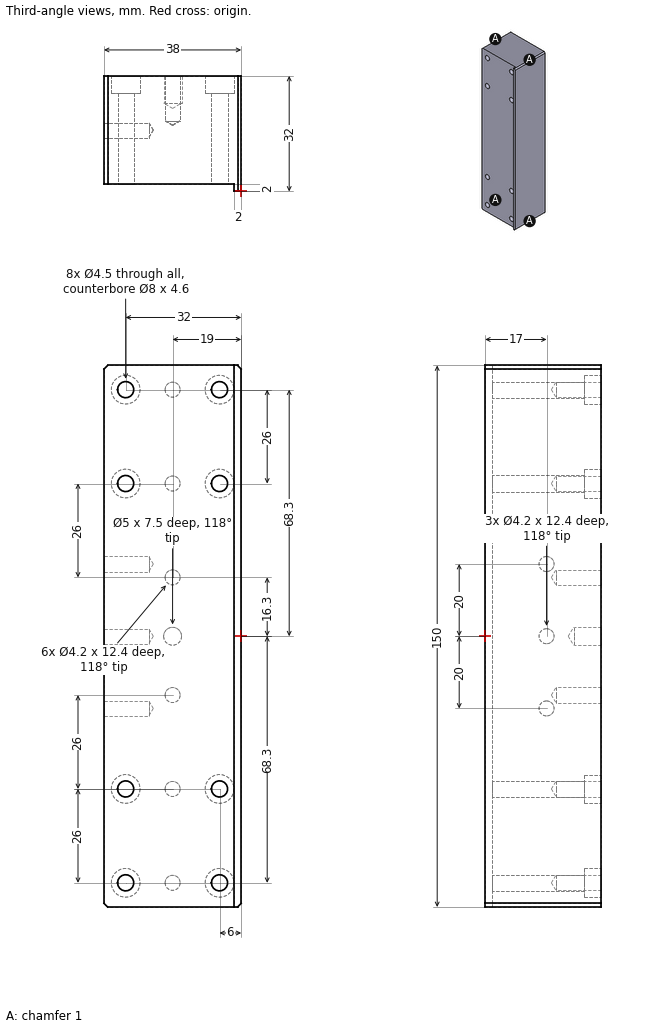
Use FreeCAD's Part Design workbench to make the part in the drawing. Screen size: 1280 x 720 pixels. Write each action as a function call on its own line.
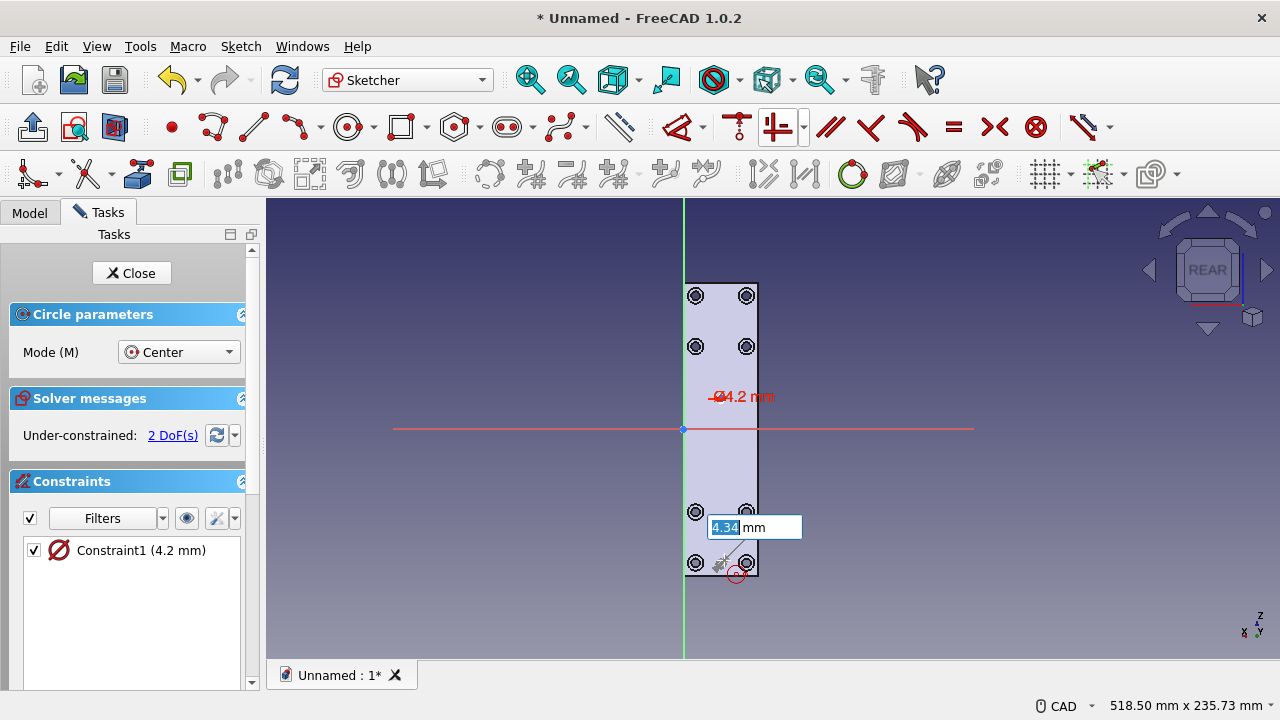
text(4.2)
key(Return)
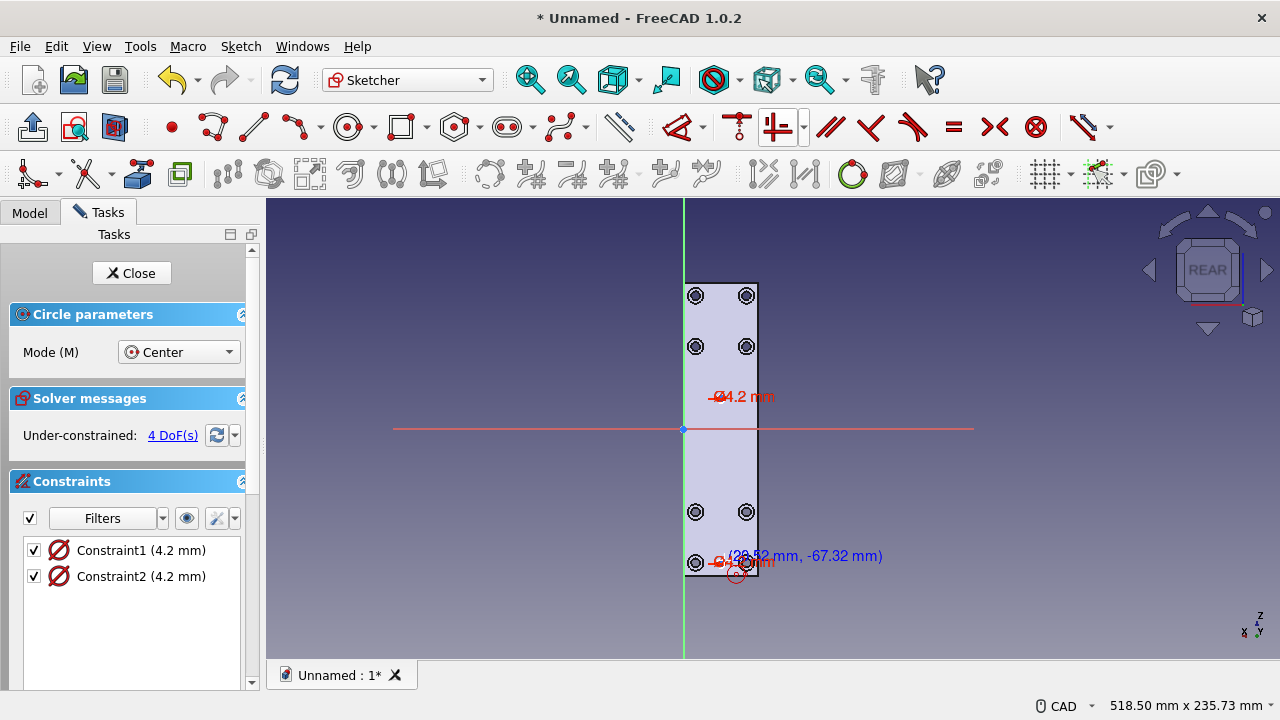
scroll(721, 512, up, 9)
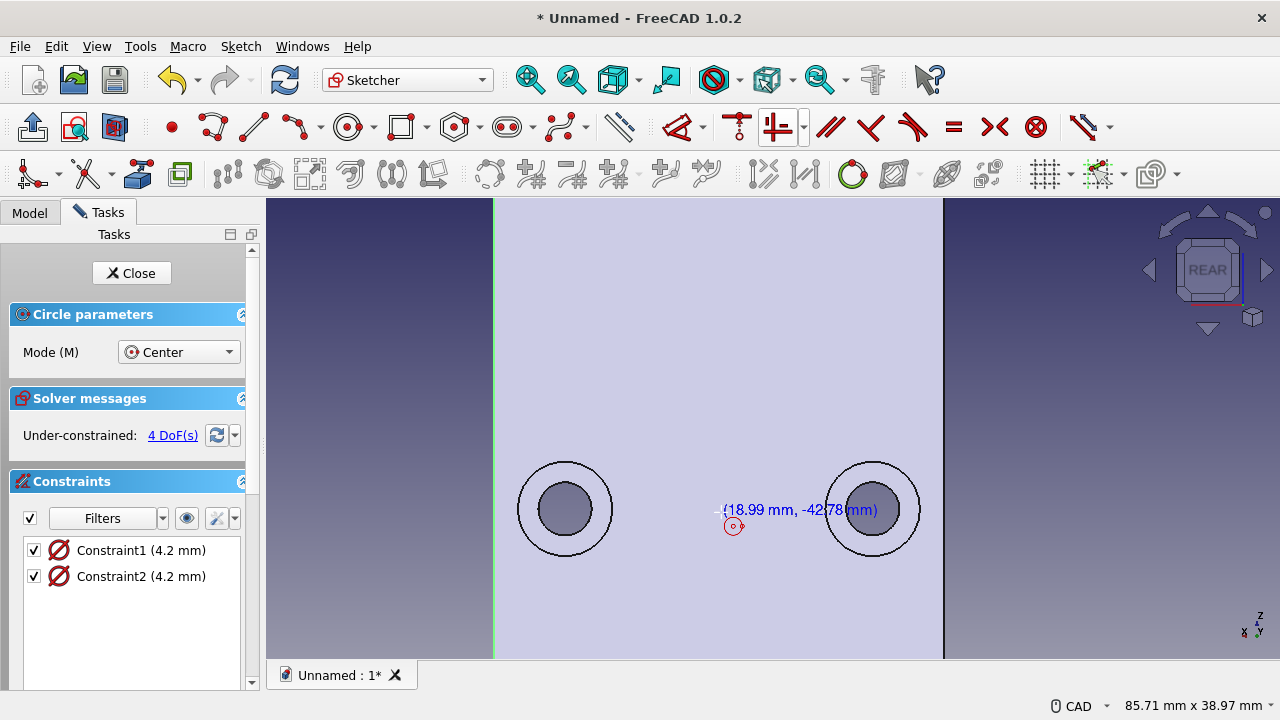
scroll(721, 512, down, 9)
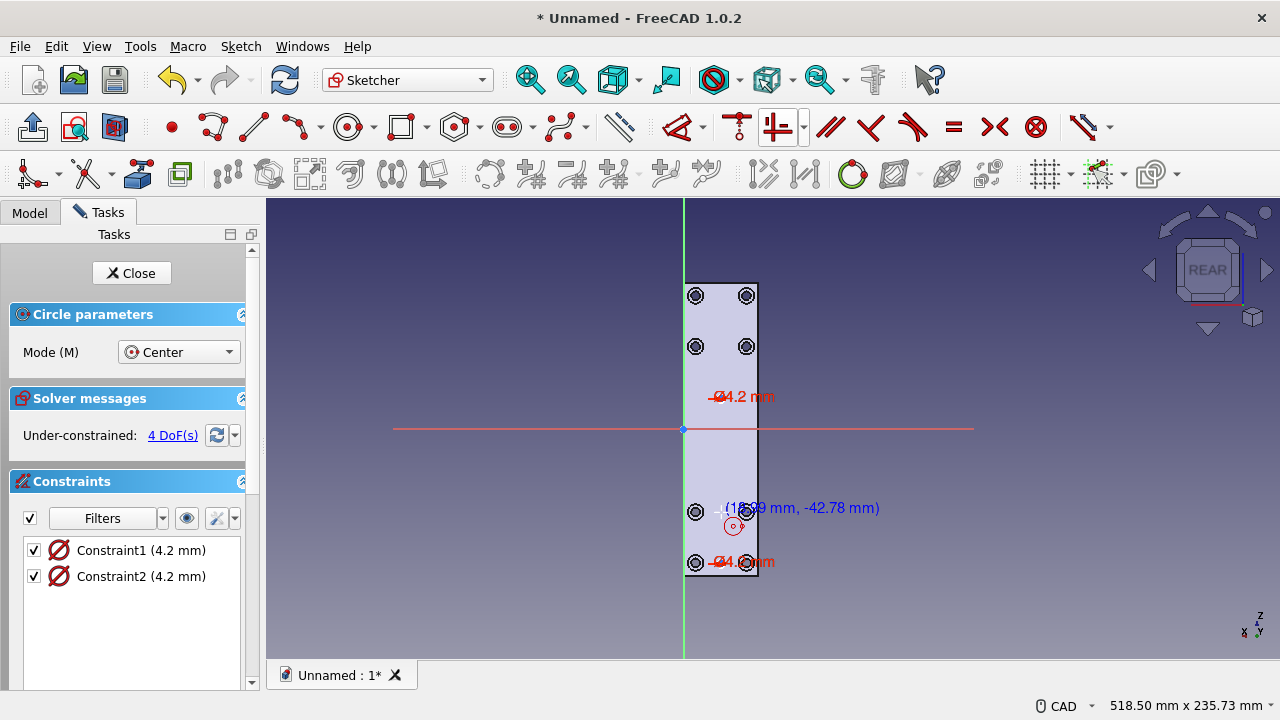
click(721, 512)
move(724, 509)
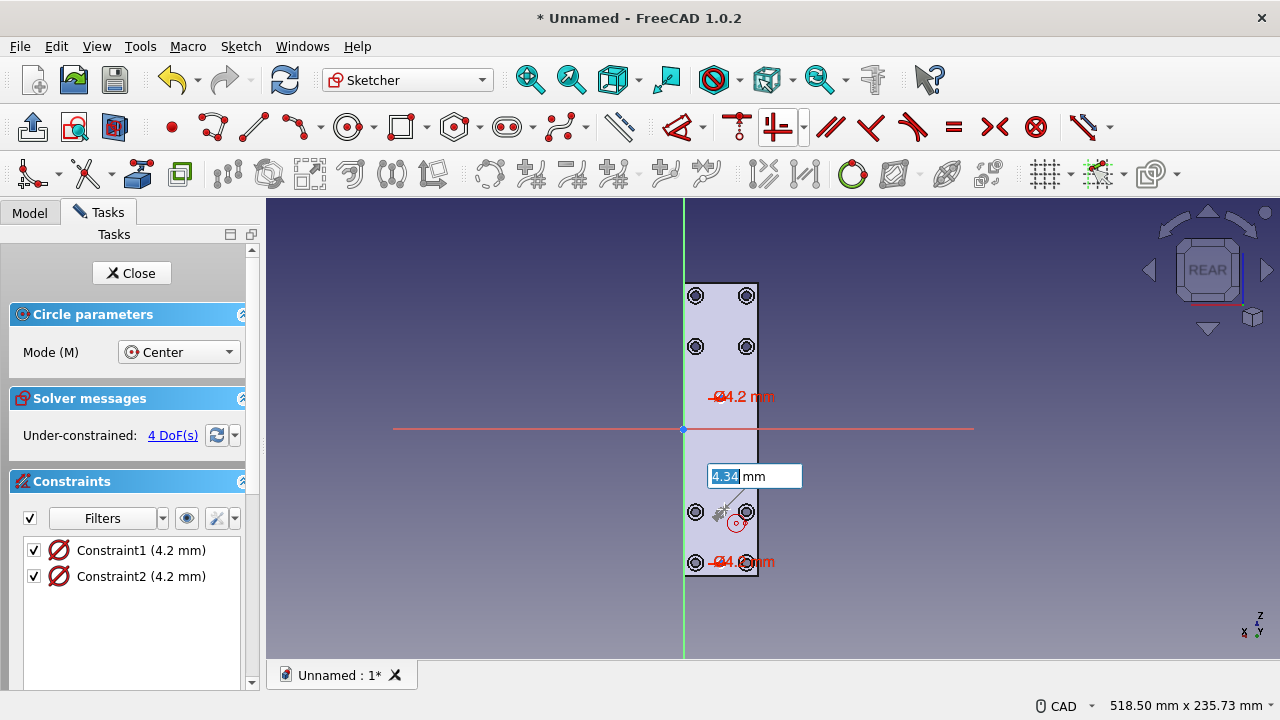
text(4.2)
key(Return)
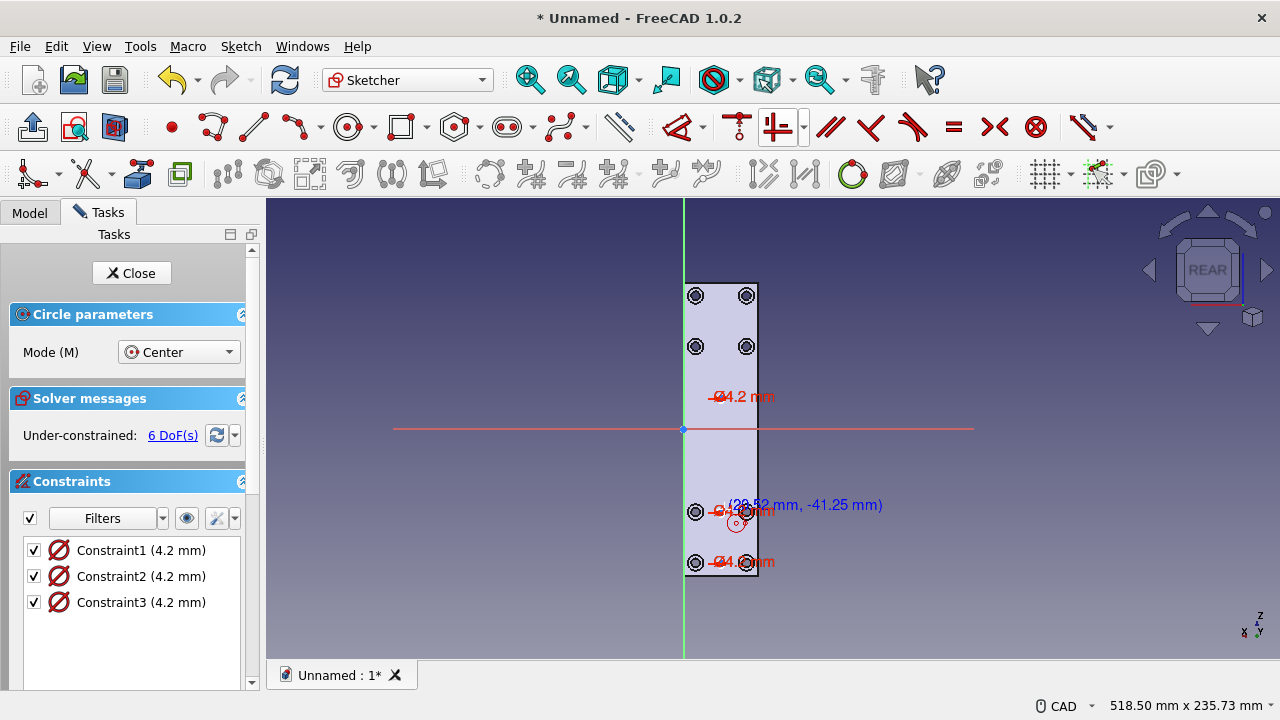
scroll(721, 347, up, 9)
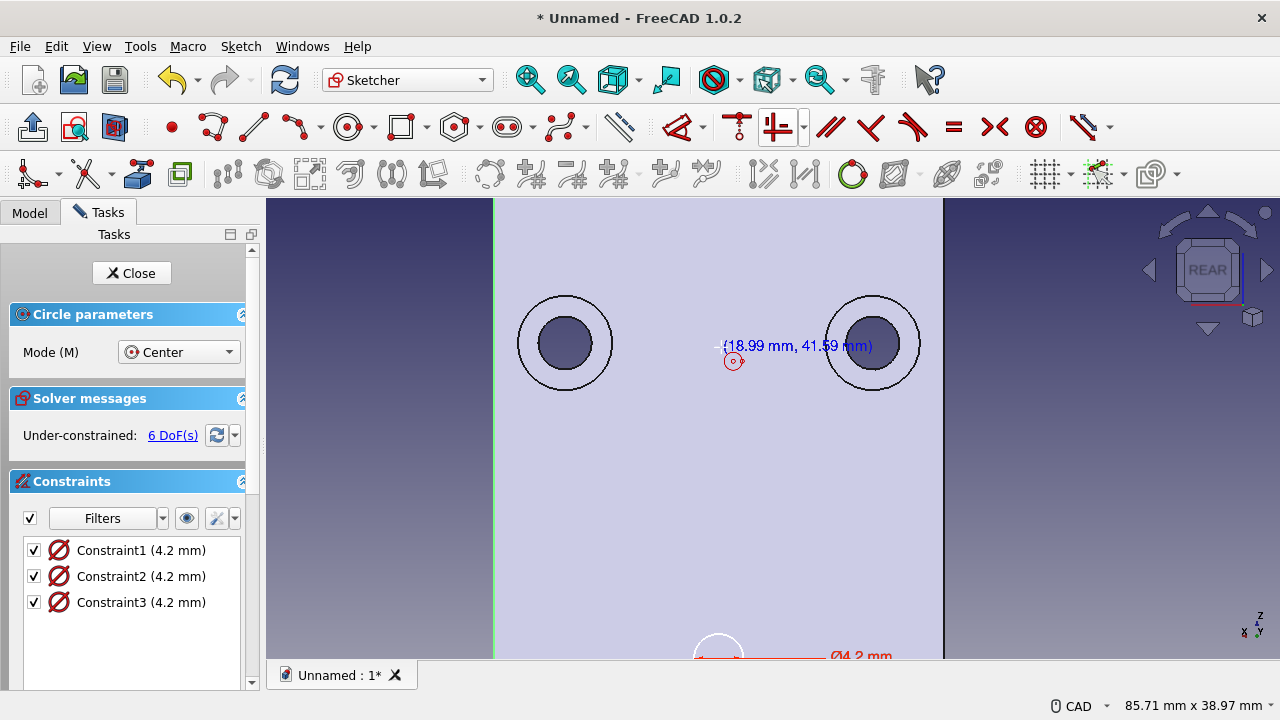
scroll(721, 346, down, 9)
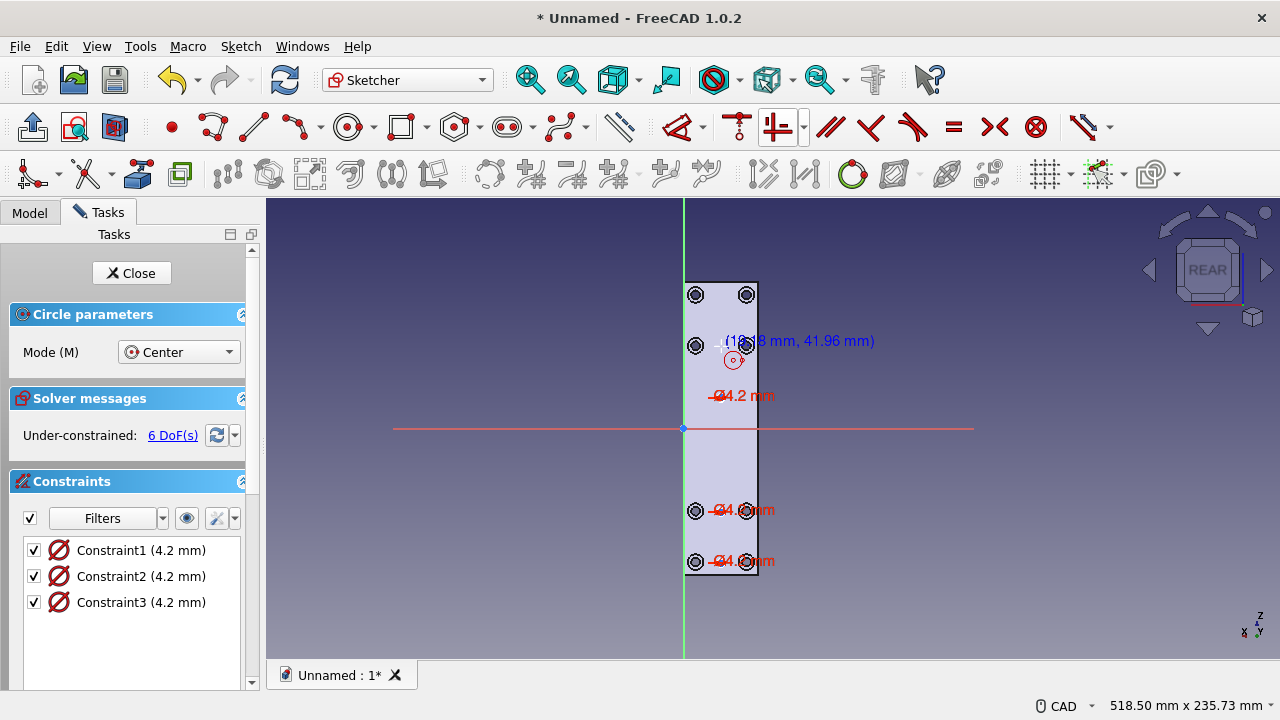
click(721, 346)
move(724, 343)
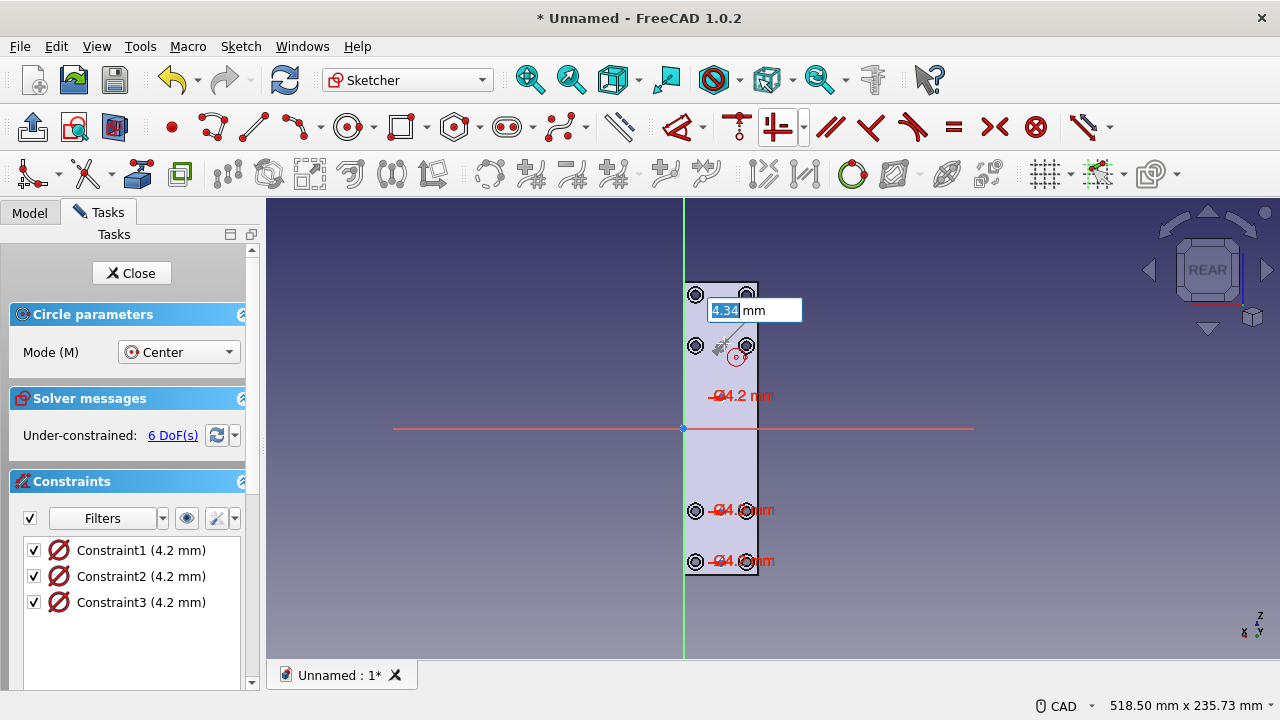
text(4.2)
key(Return)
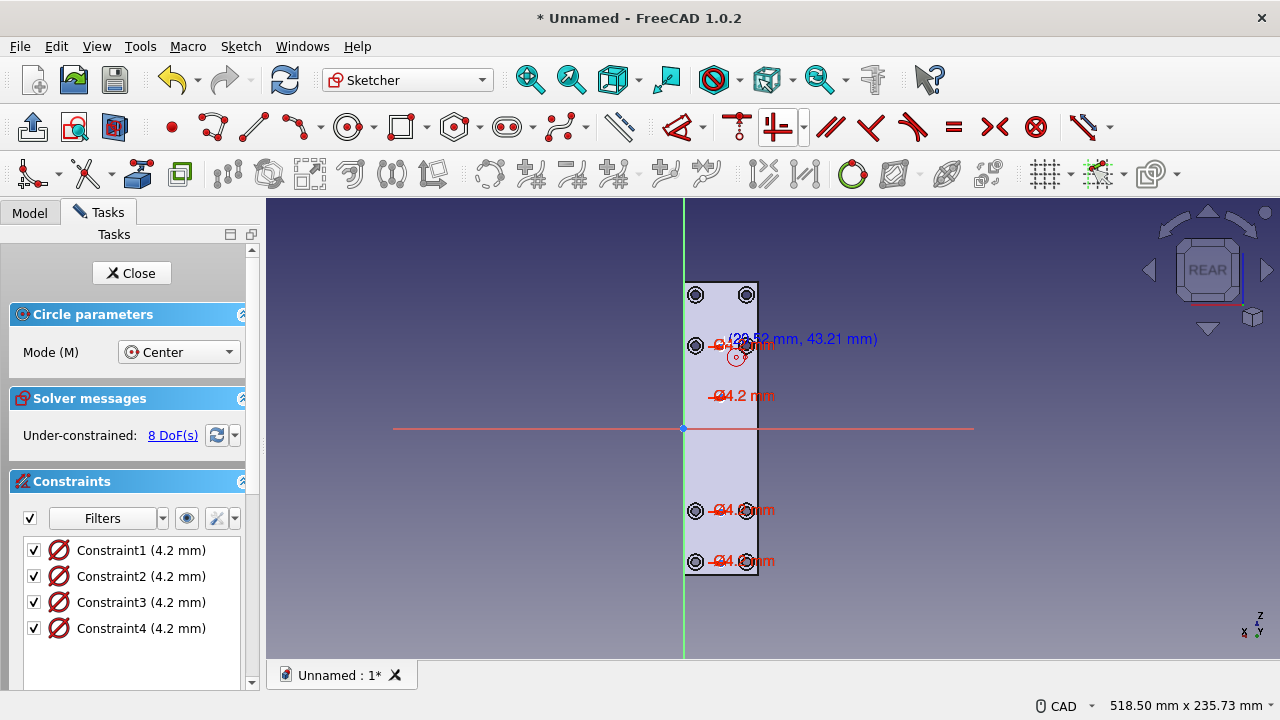
scroll(721, 295, up, 9)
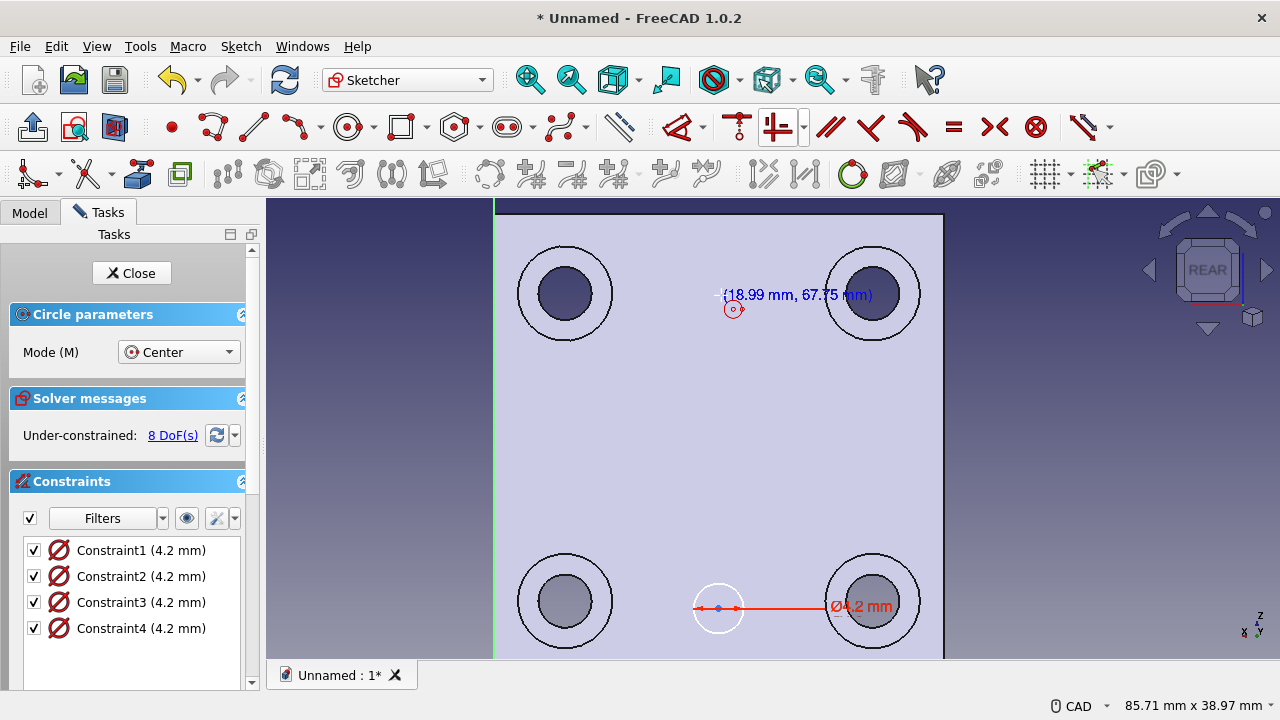
scroll(721, 295, down, 9)